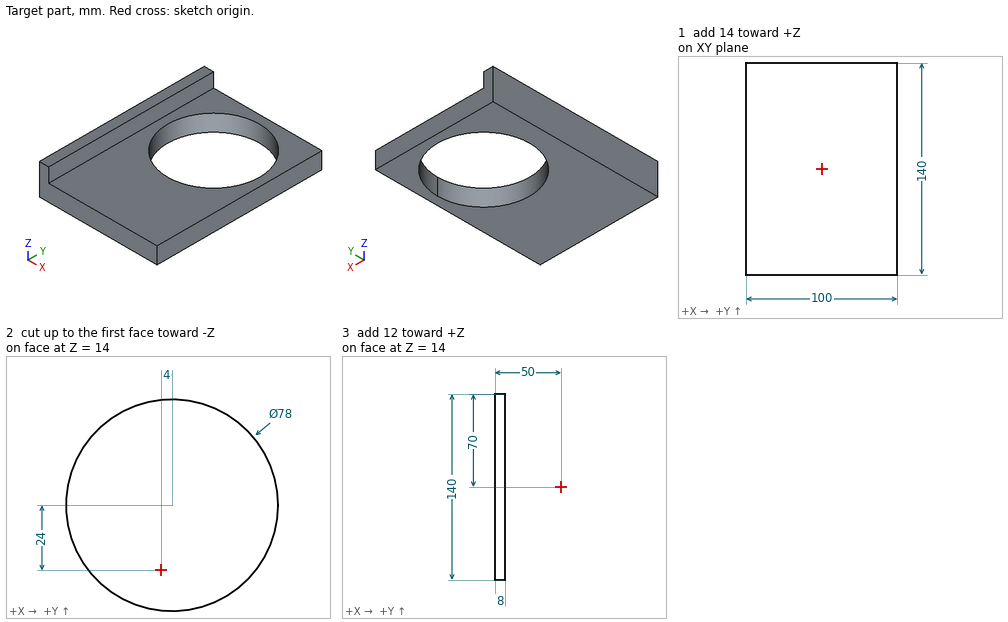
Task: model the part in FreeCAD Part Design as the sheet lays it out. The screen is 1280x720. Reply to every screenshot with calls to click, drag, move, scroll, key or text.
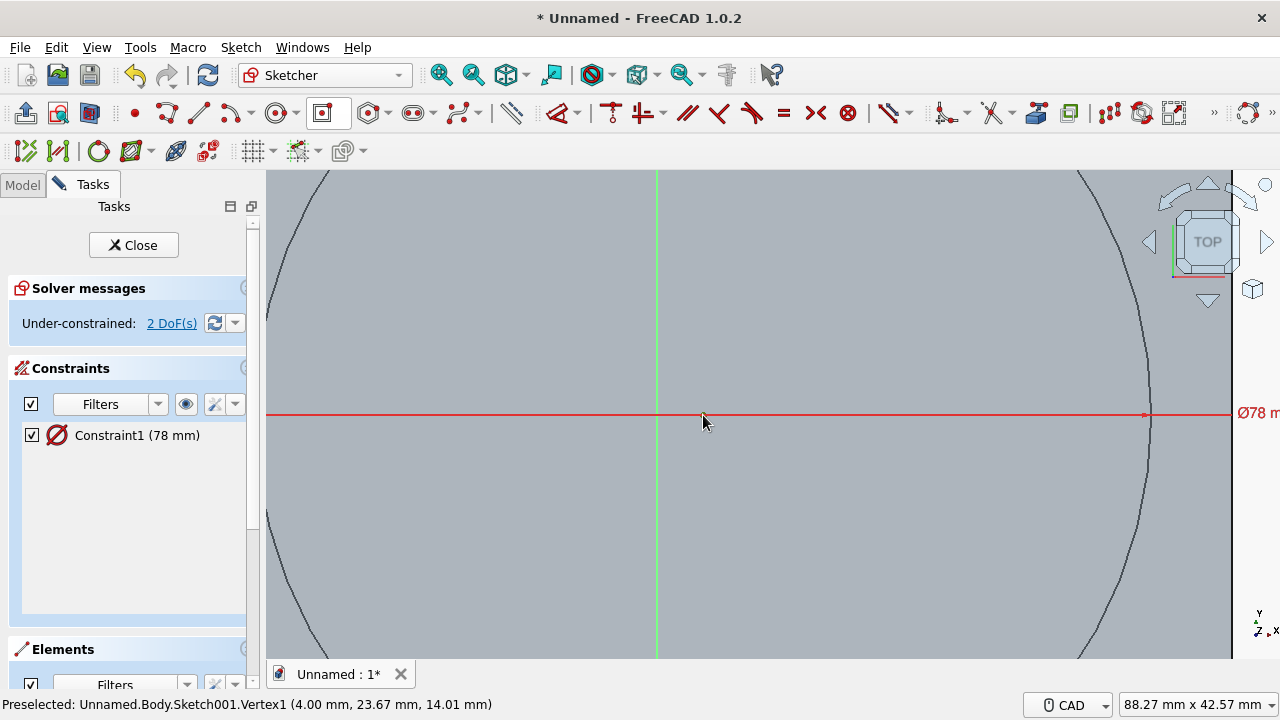
click(580, 114)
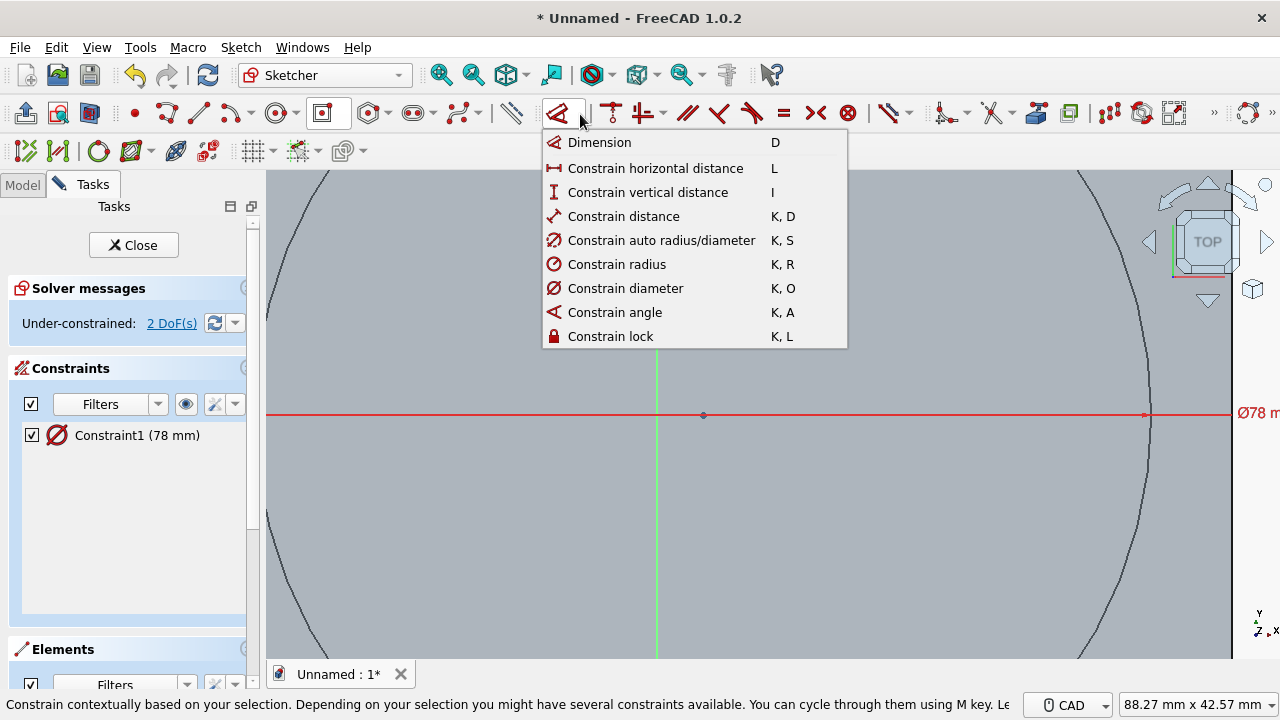
click(695, 168)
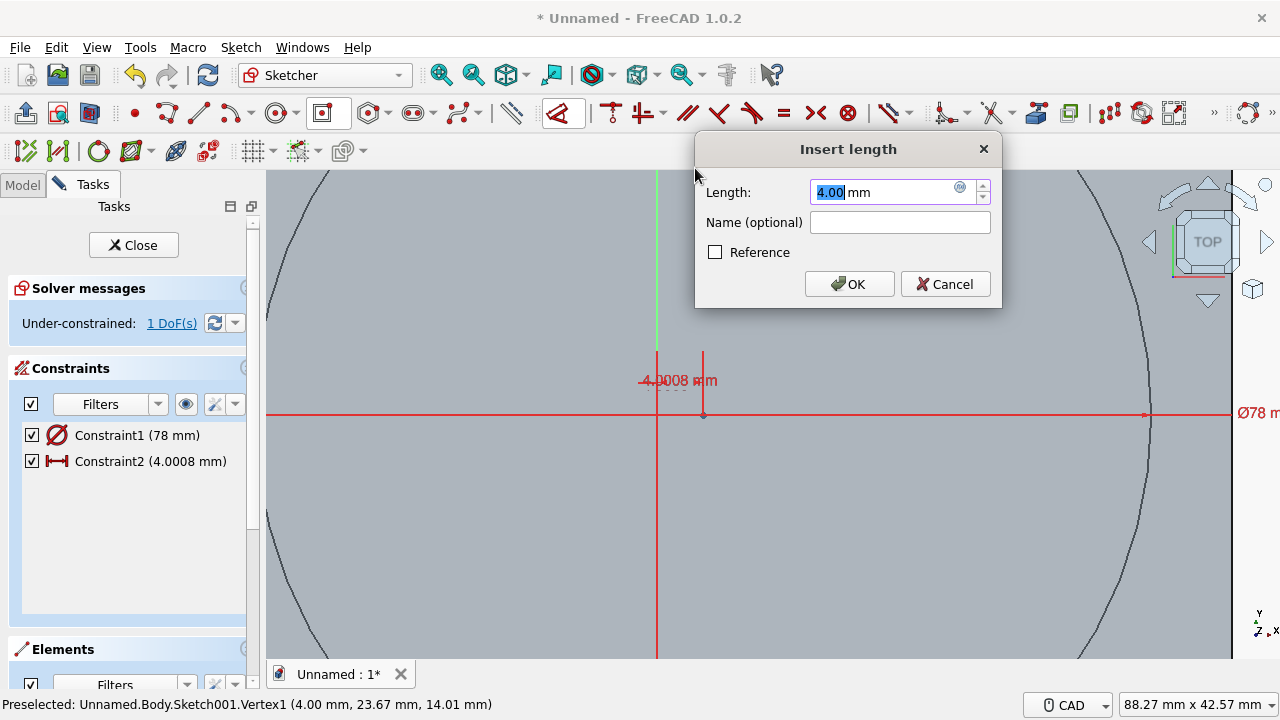
text(4)
key(Return)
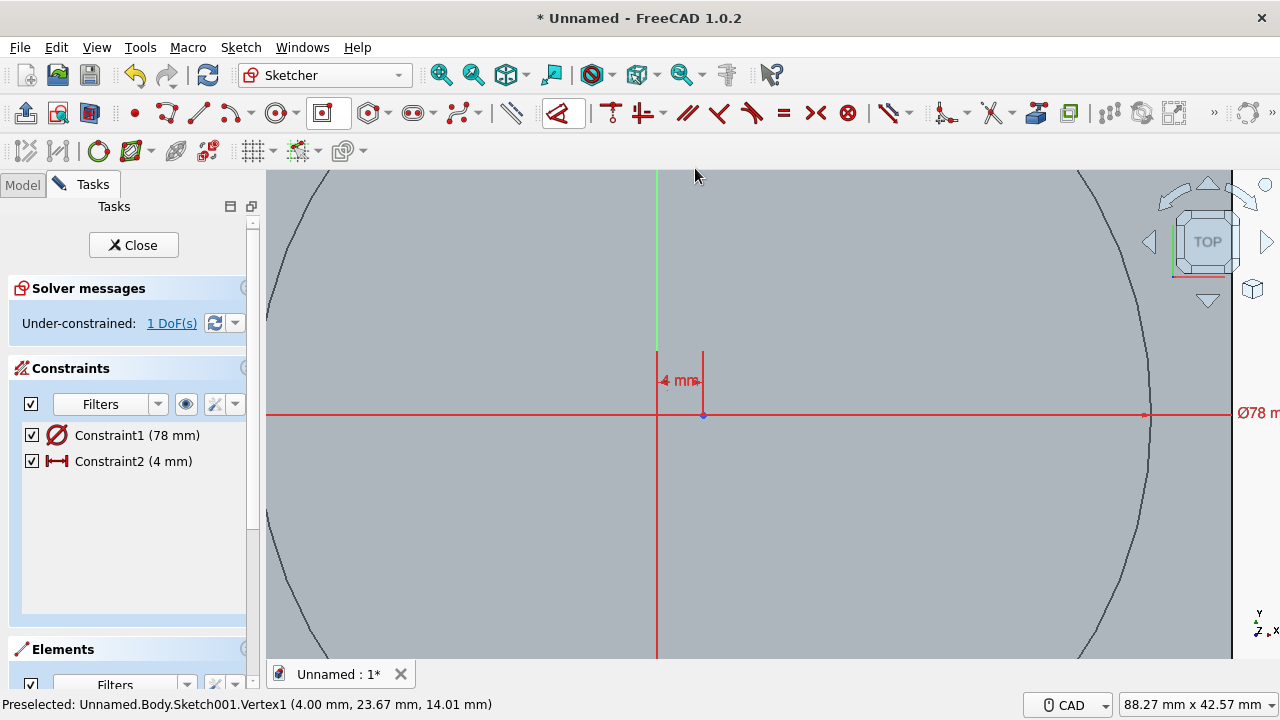
click(703, 415)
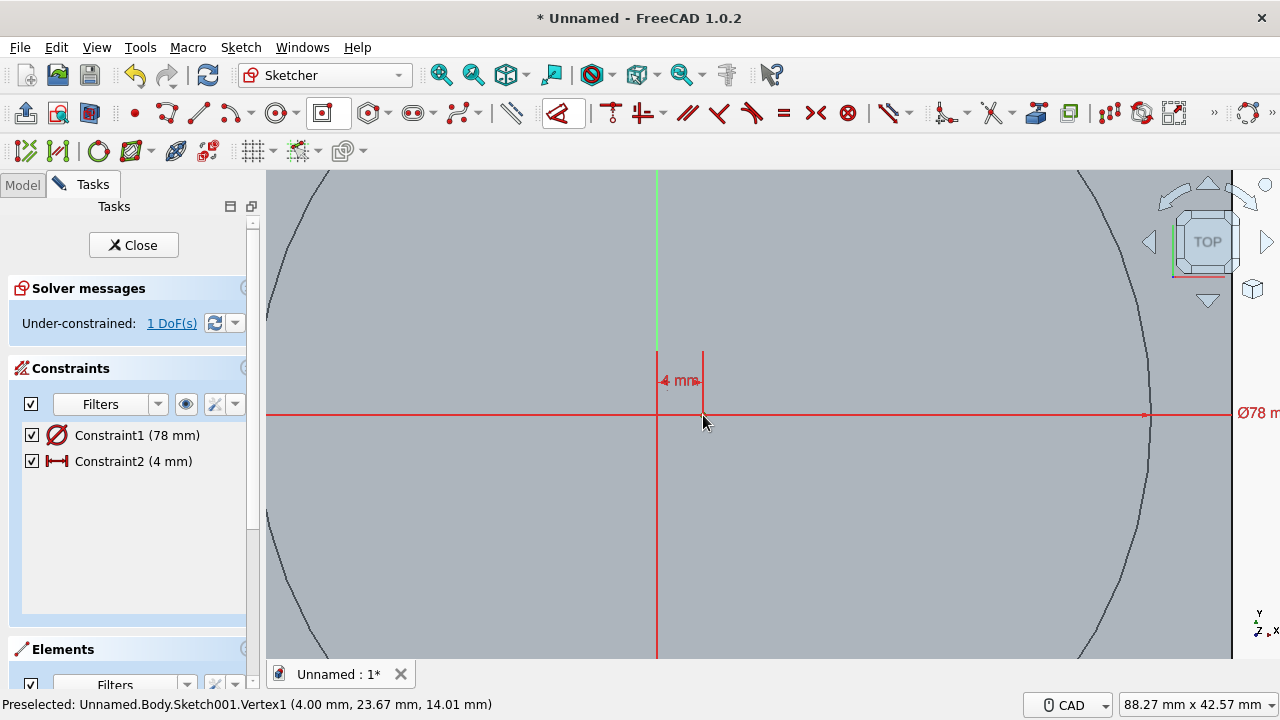
key(i)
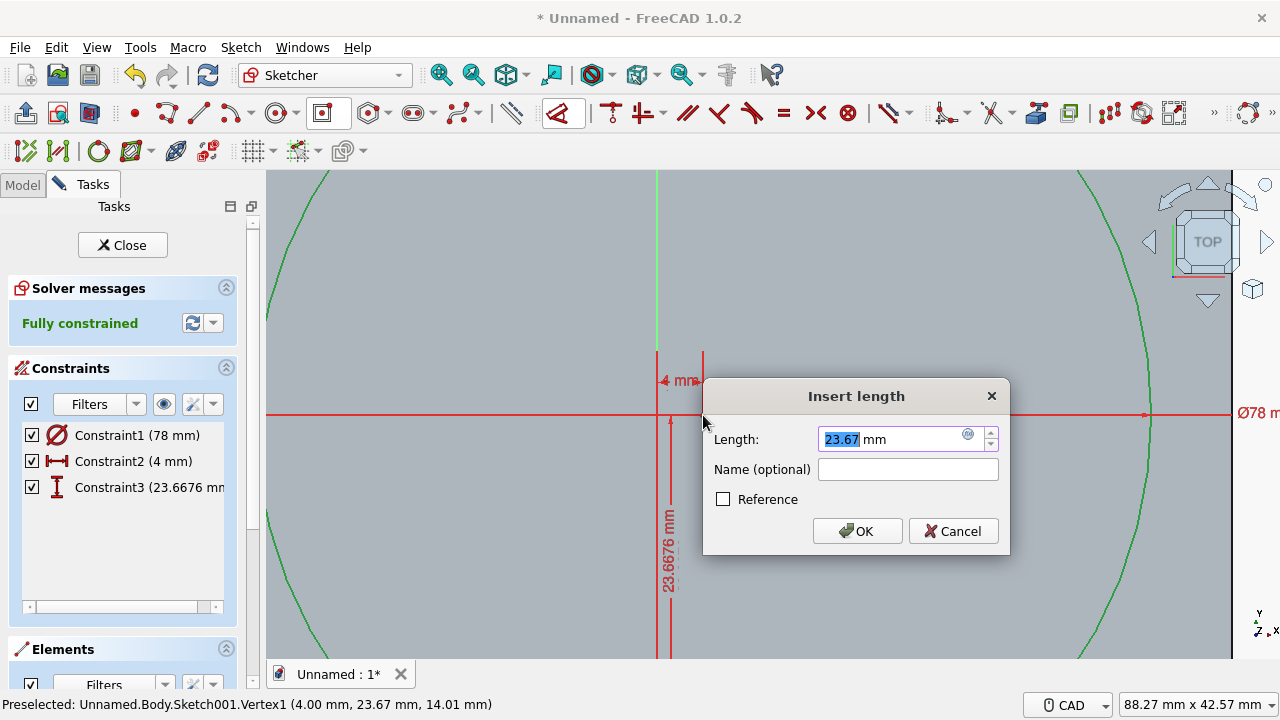
text(24)
key(Return)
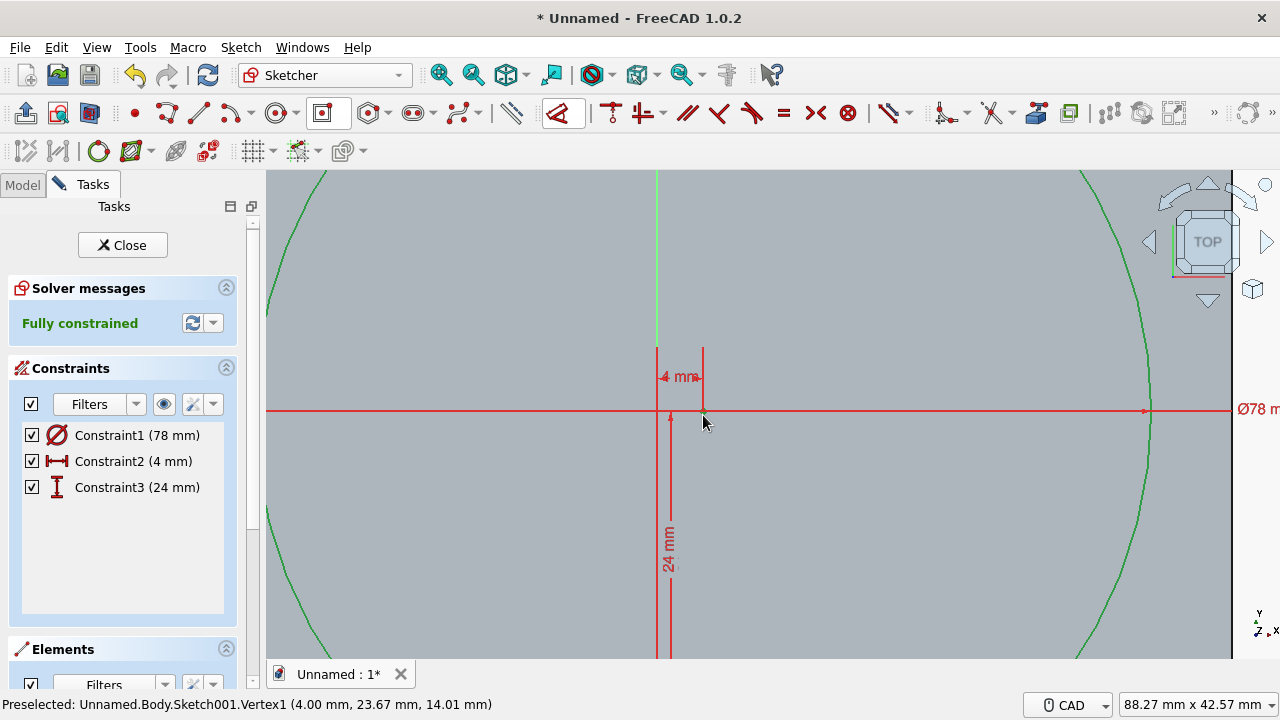
click(123, 245)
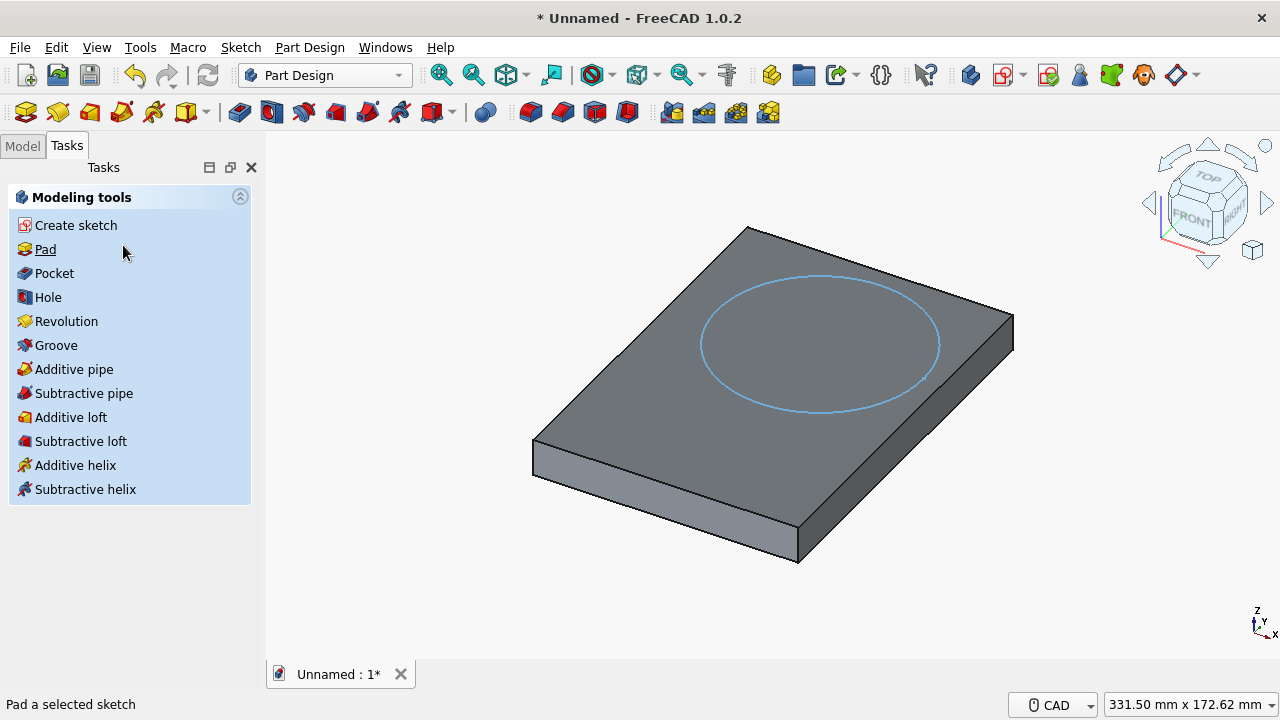
click(240, 112)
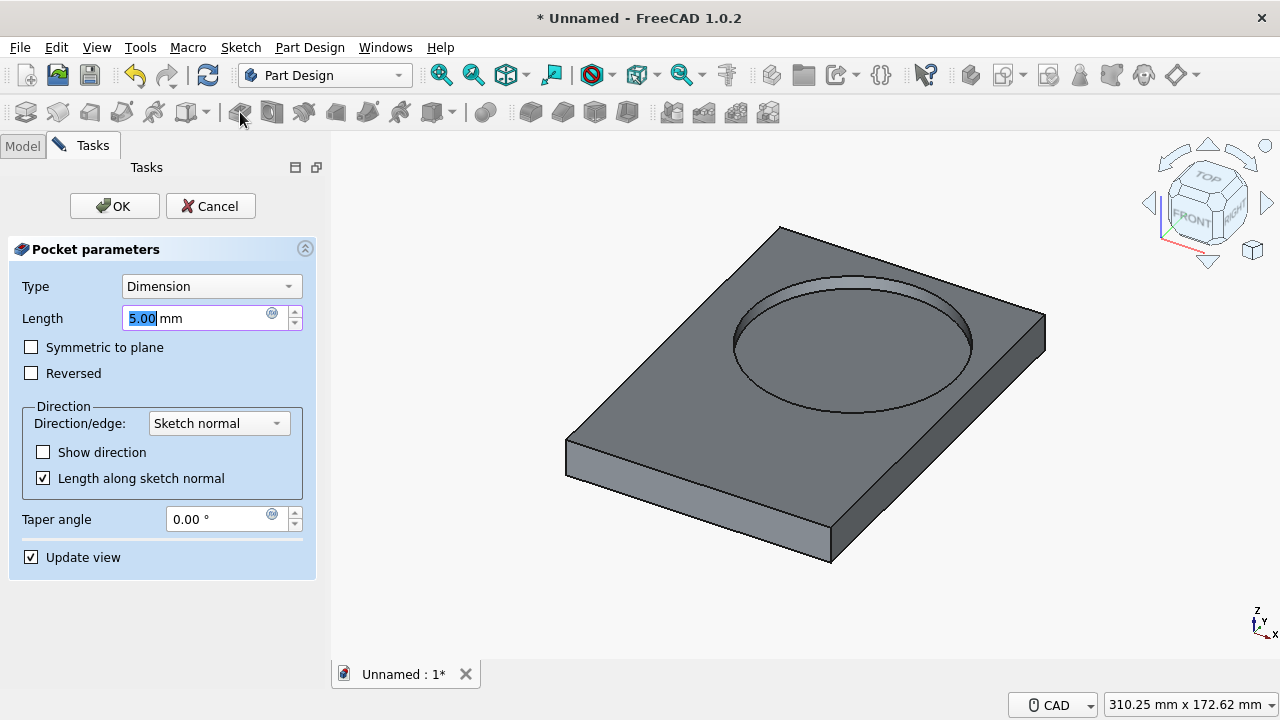
click(212, 286)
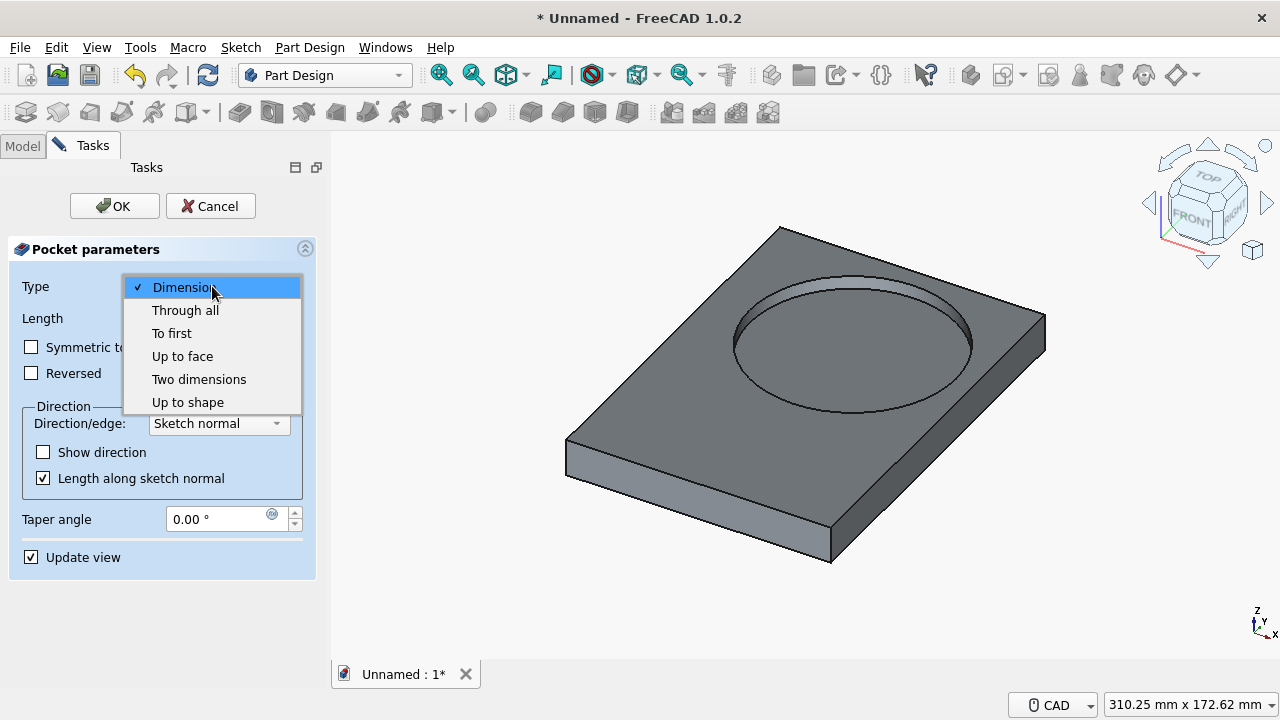
click(212, 334)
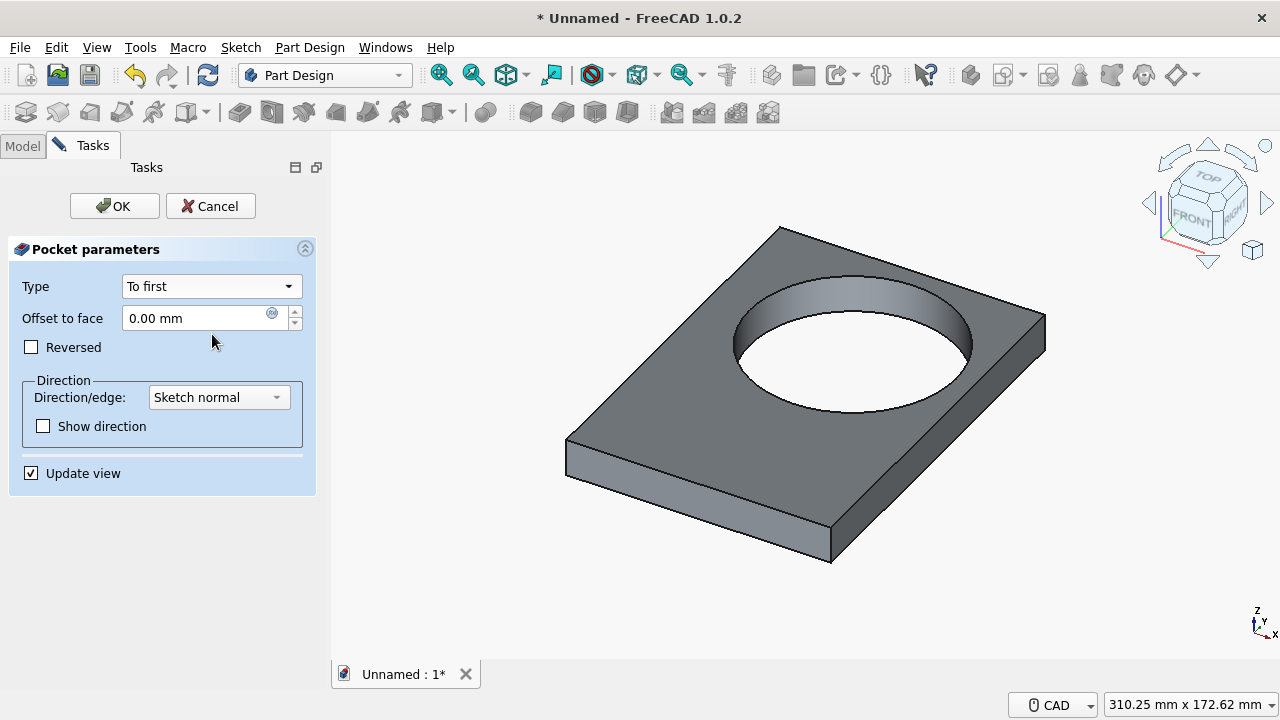
click(115, 206)